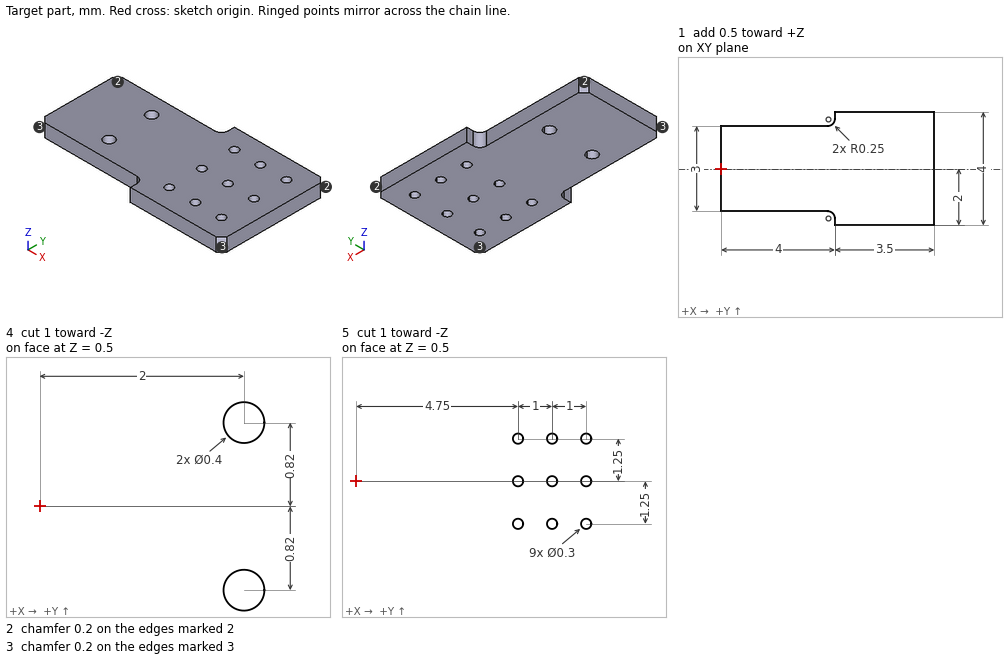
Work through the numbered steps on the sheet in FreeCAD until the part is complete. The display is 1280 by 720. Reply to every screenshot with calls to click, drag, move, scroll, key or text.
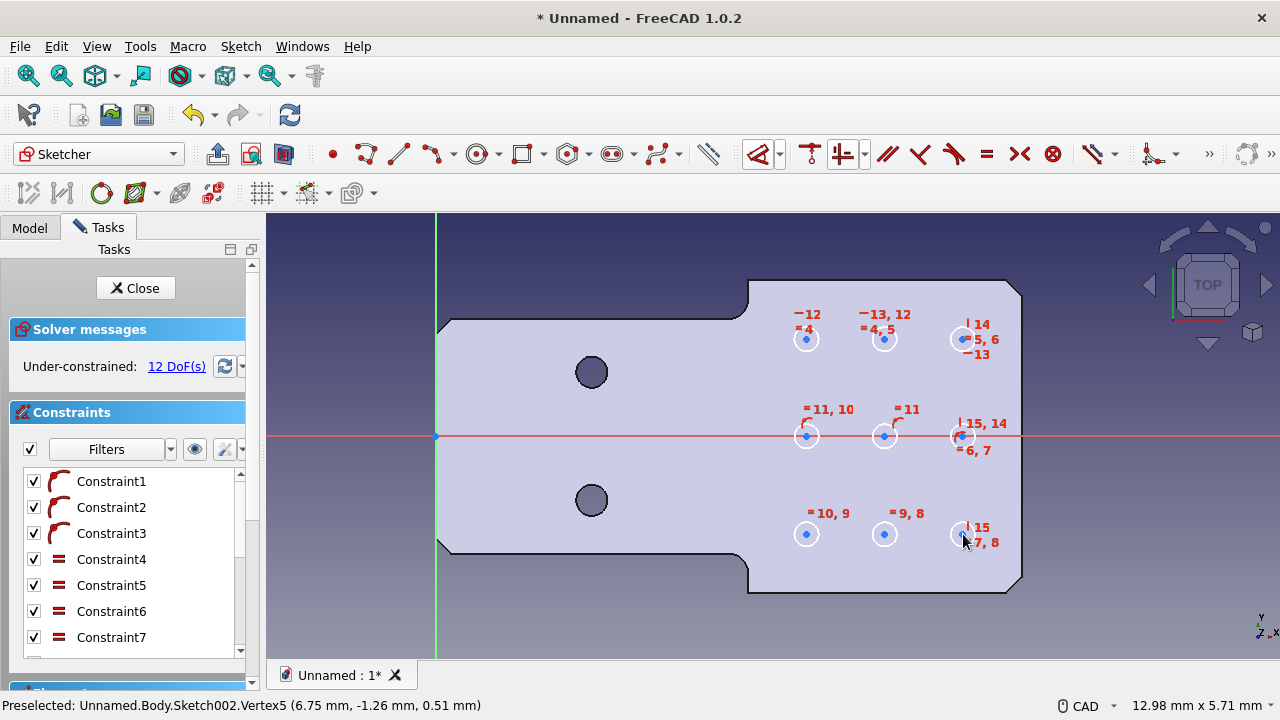
click(885, 339)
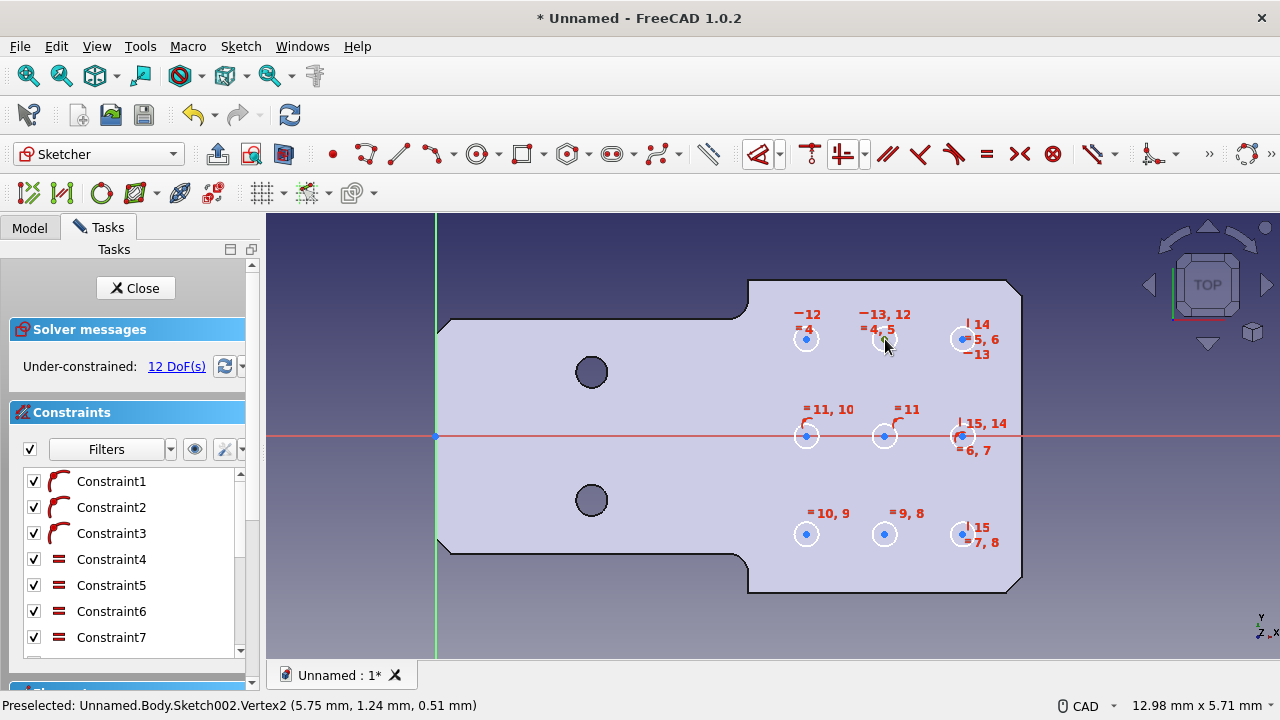
click(885, 534)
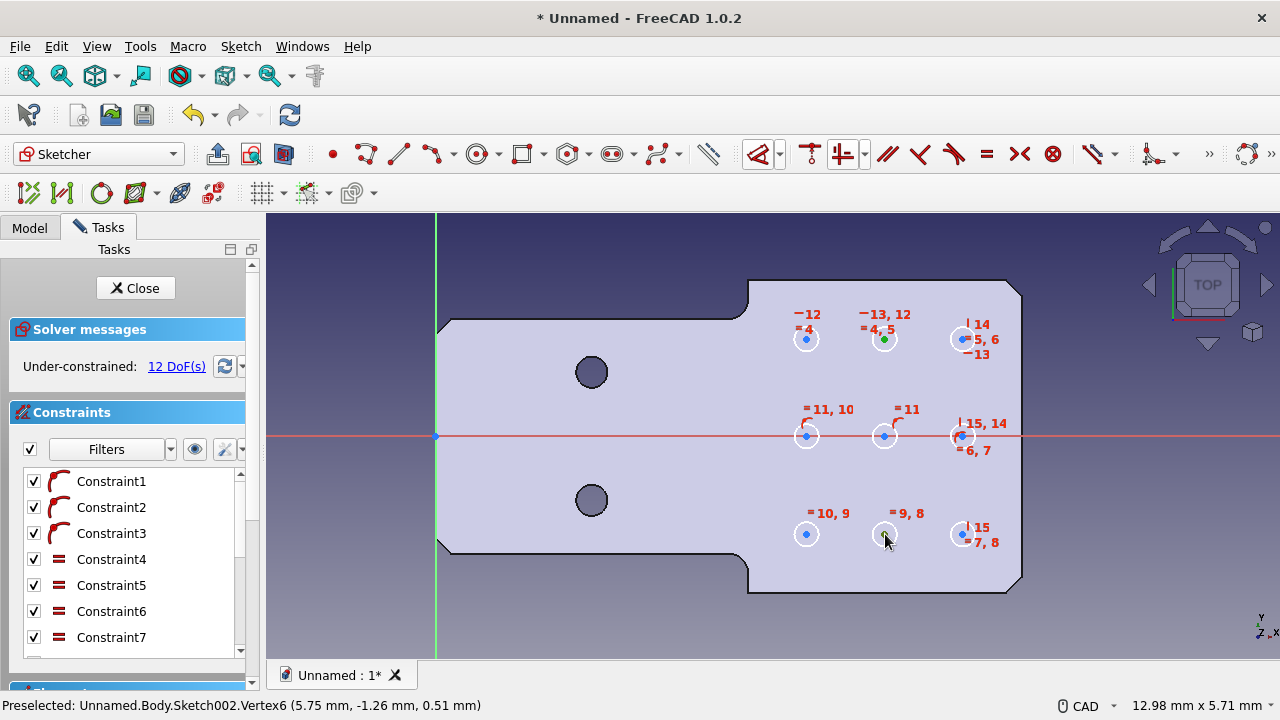
key(v)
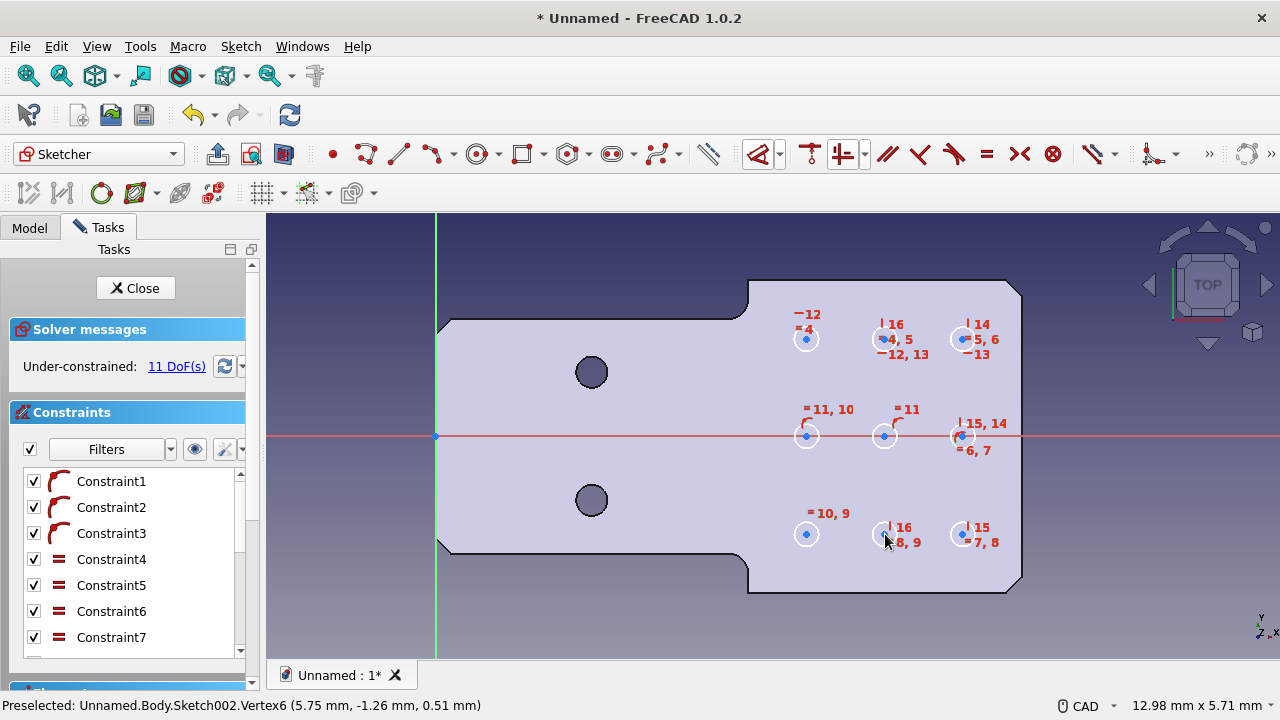
click(961, 536)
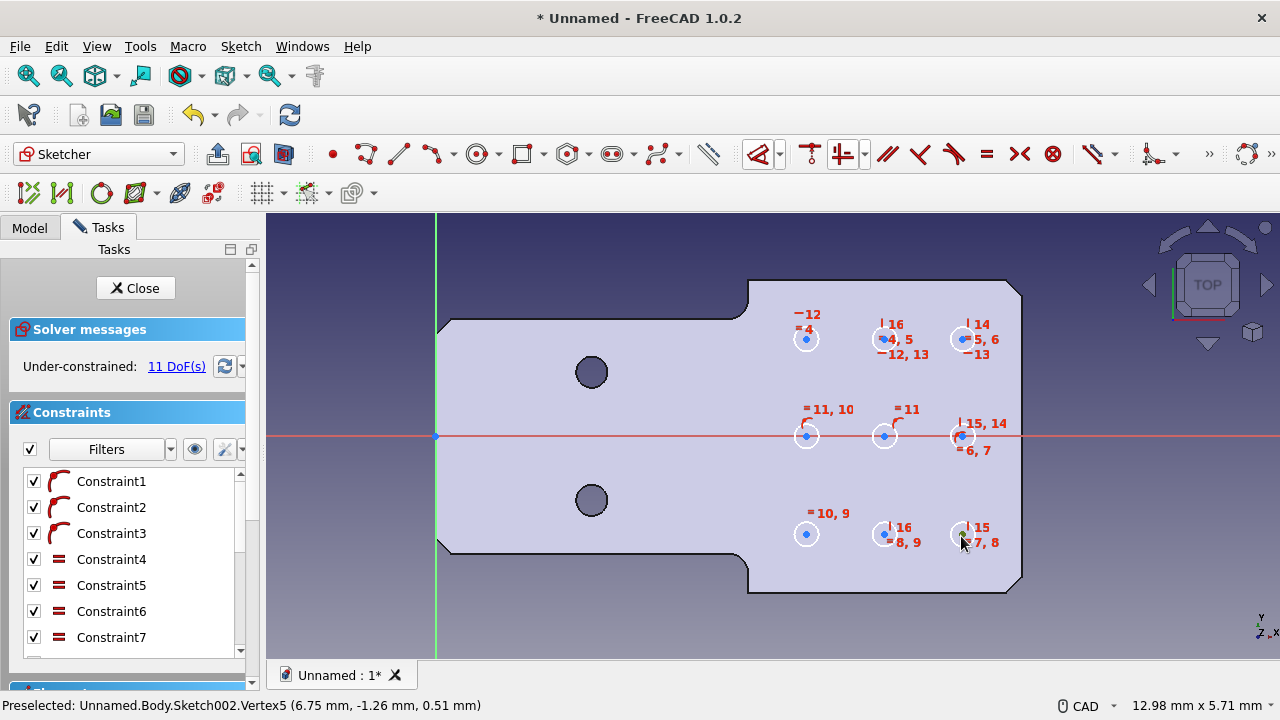
click(883, 536)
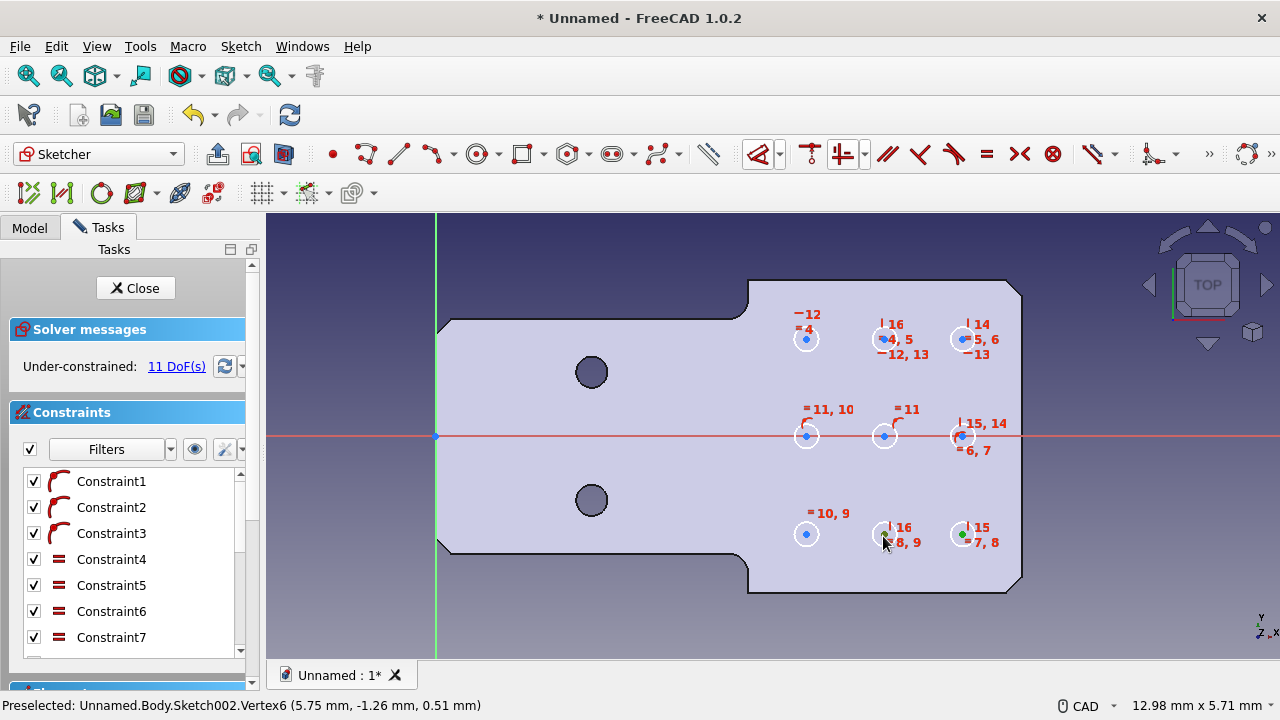
click(864, 154)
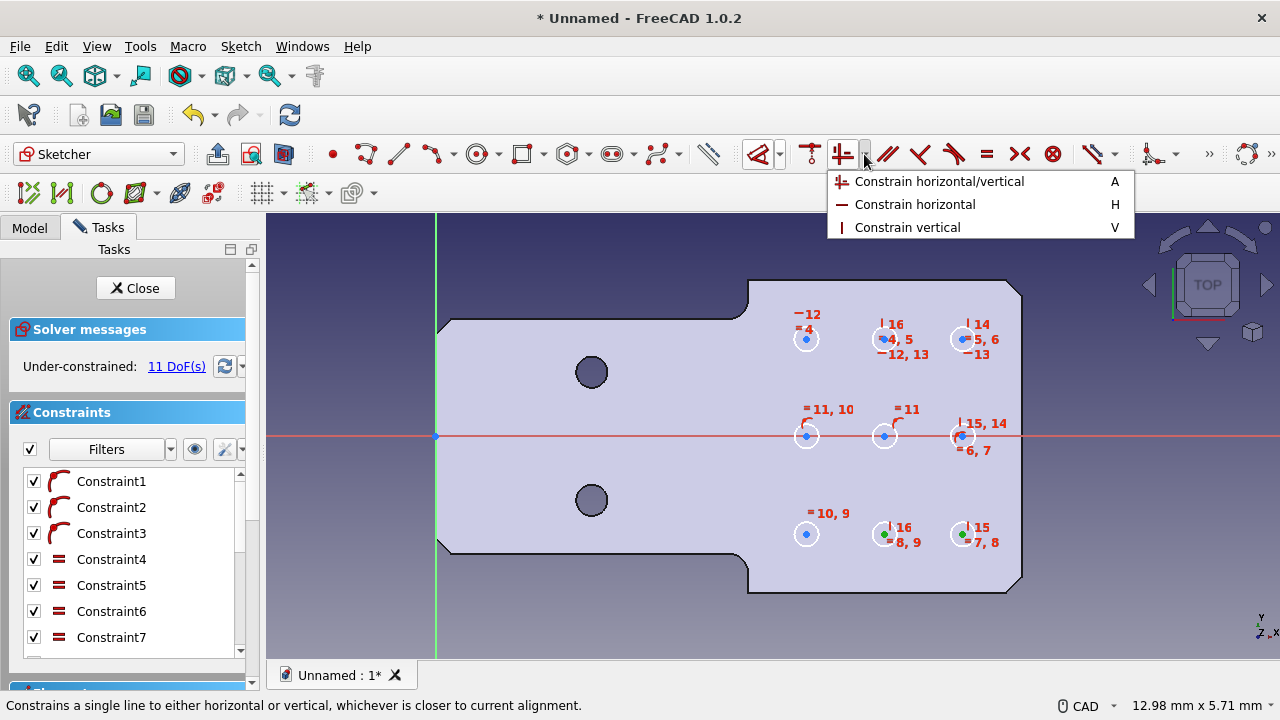
click(981, 204)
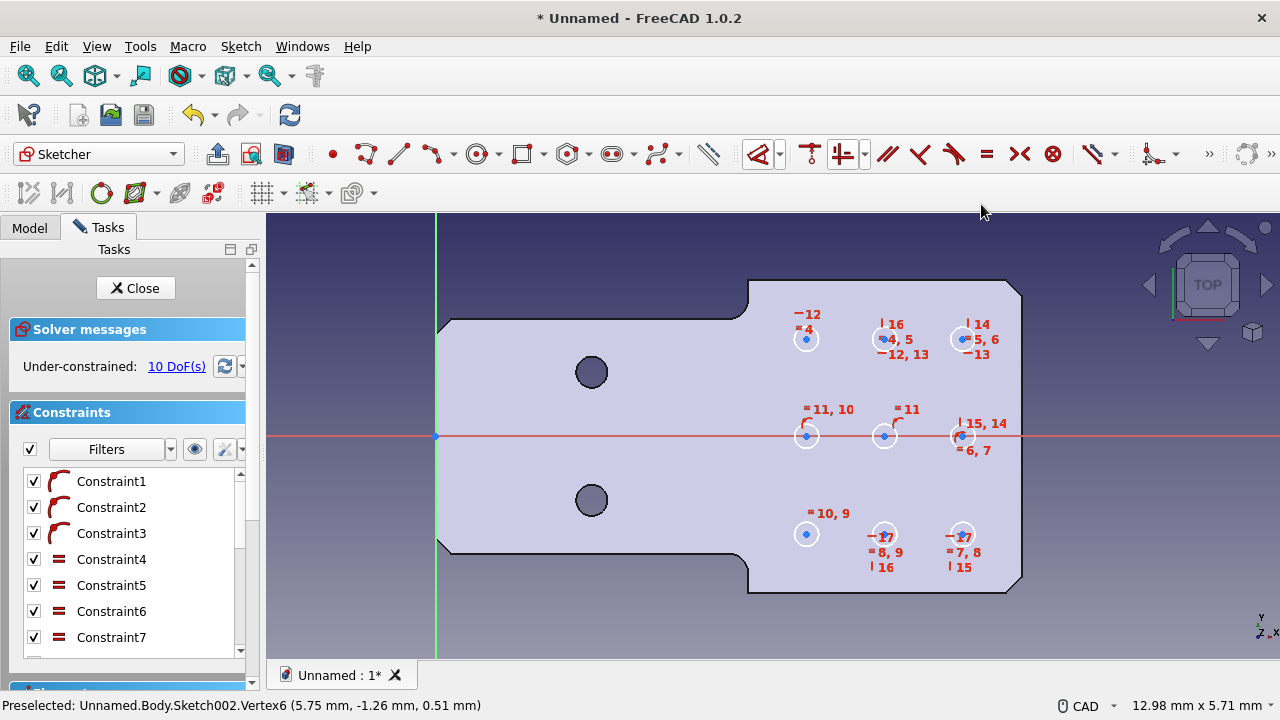
click(806, 339)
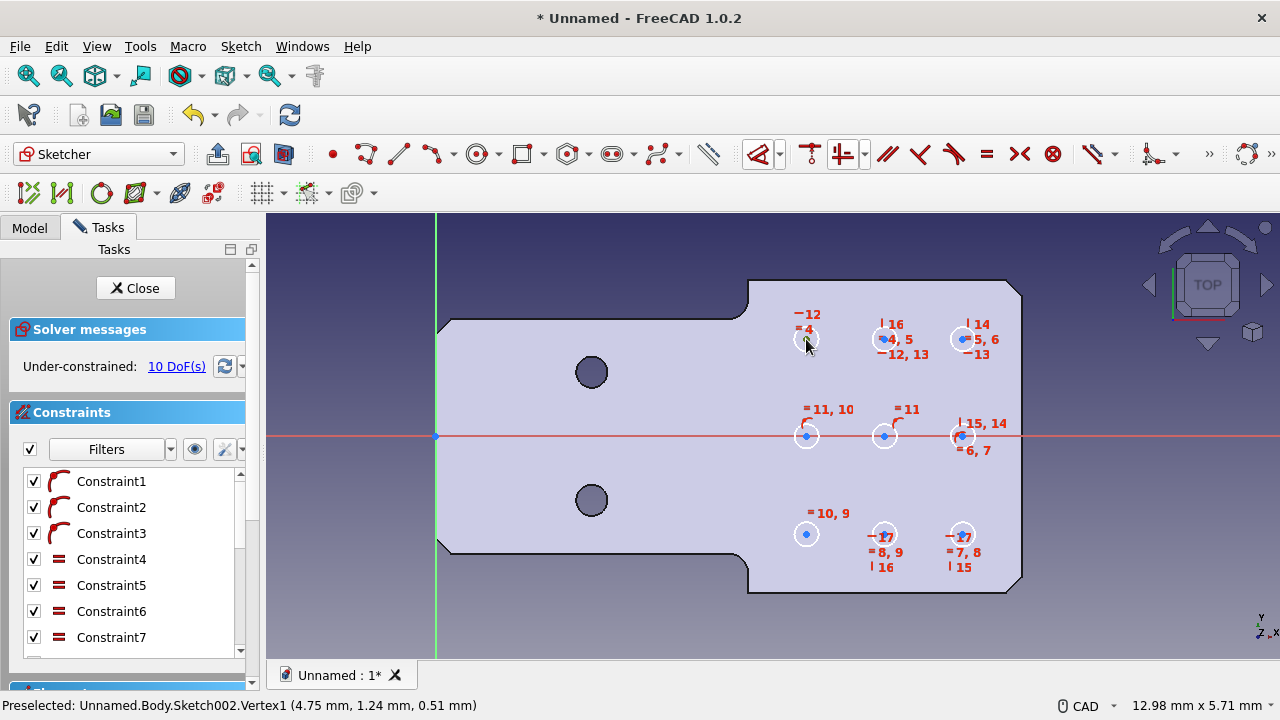
click(807, 534)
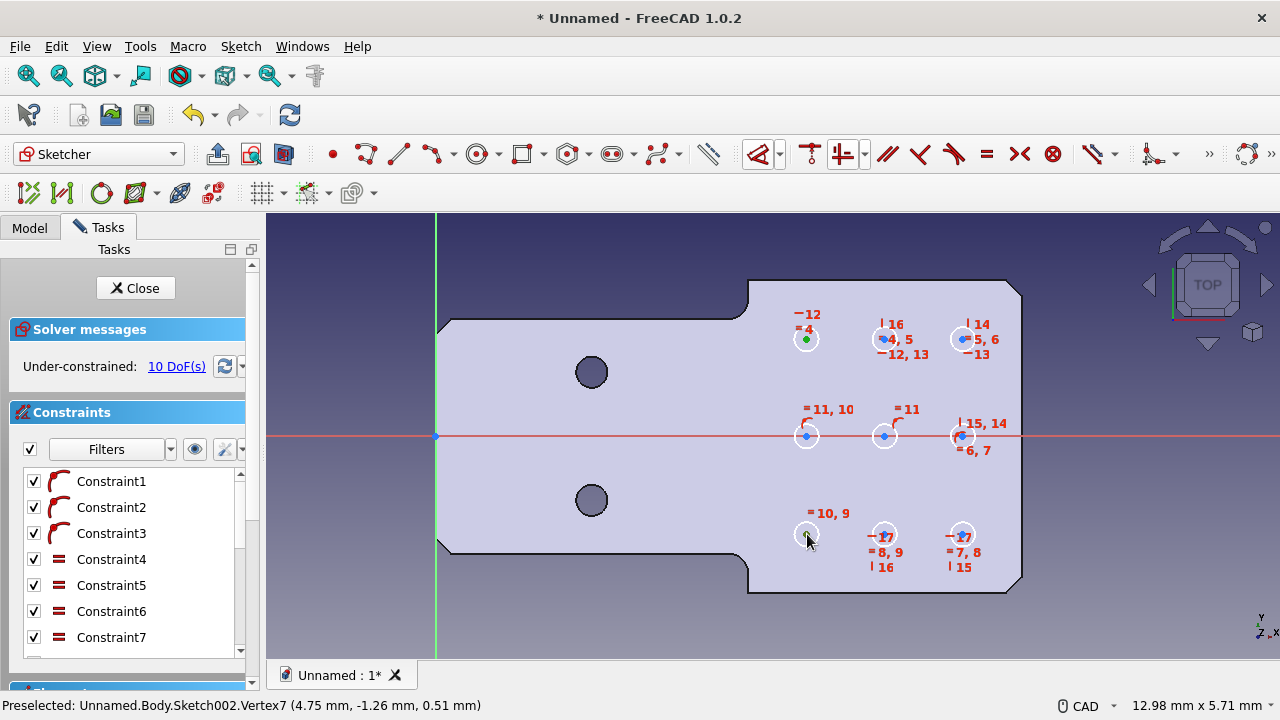
key(v)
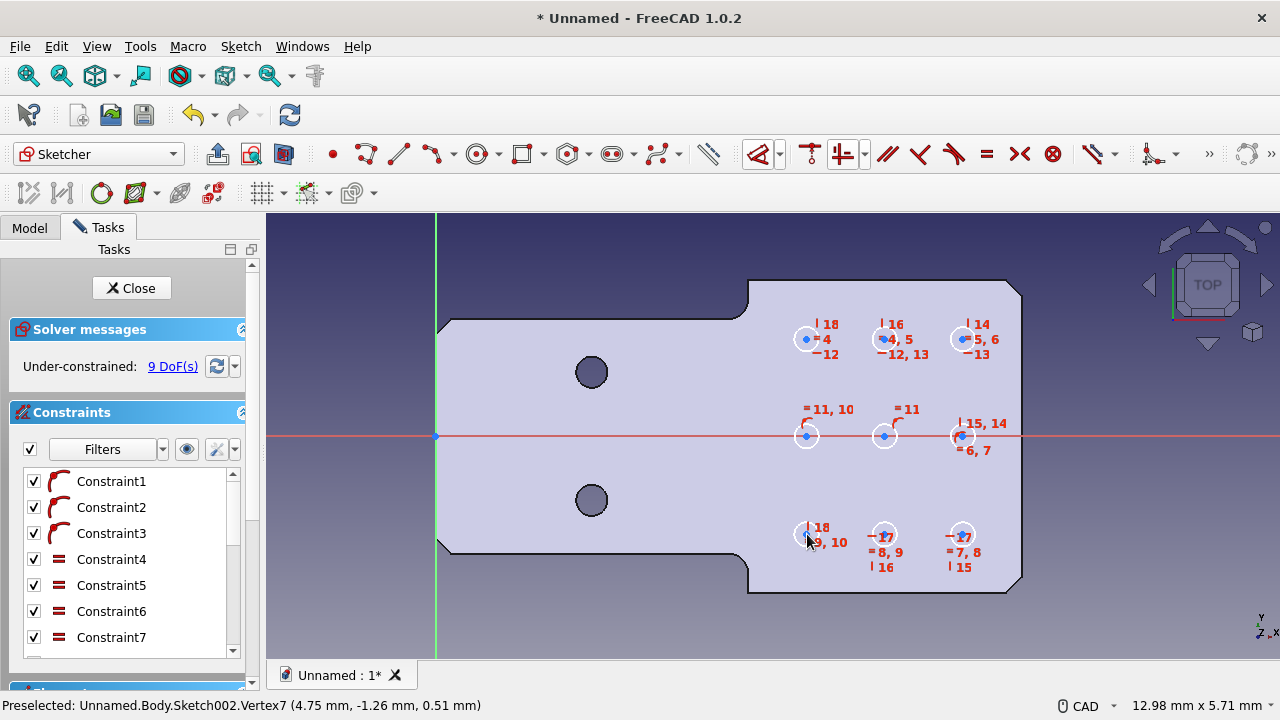
scroll(885, 534, up, 4)